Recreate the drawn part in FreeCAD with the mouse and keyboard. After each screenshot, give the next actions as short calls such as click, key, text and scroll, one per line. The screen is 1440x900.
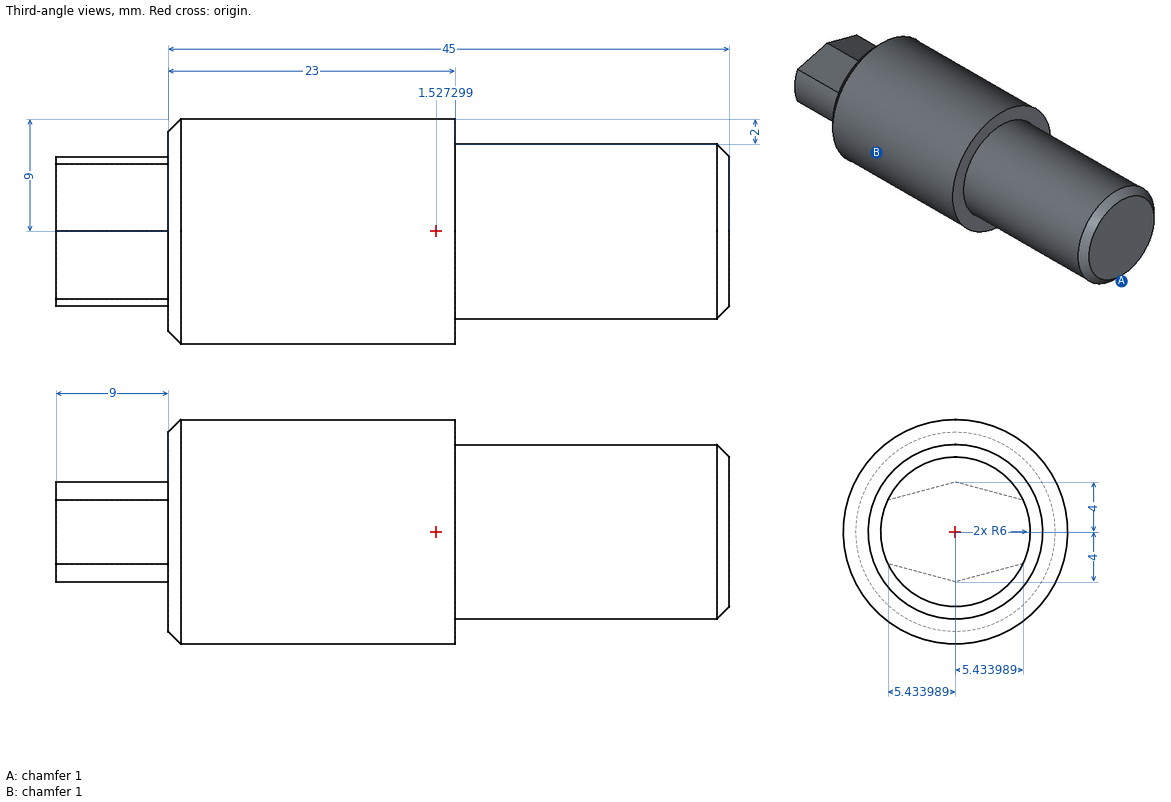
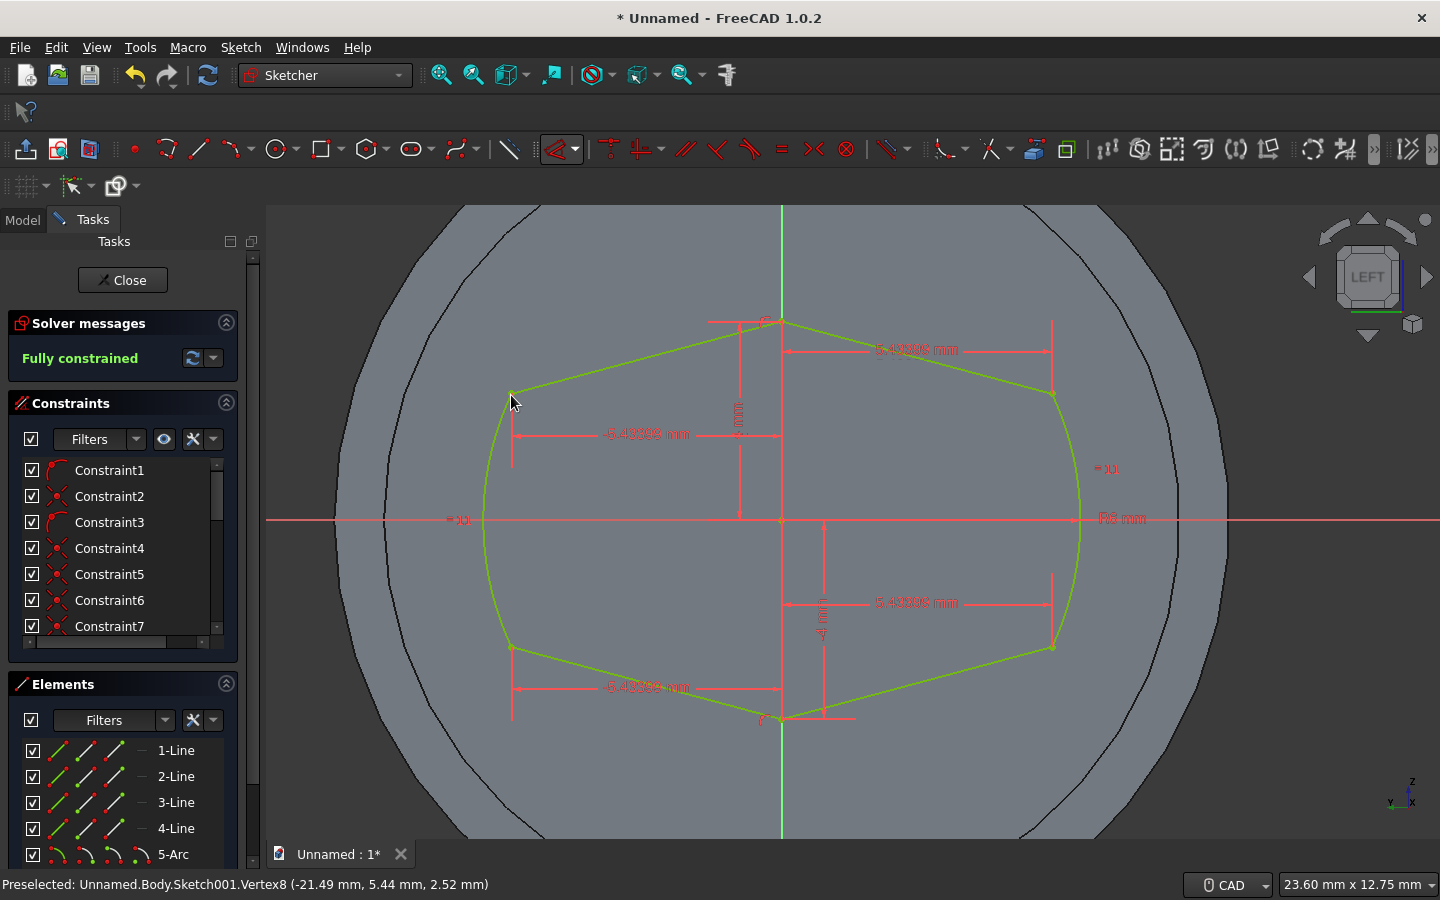
click(123, 280)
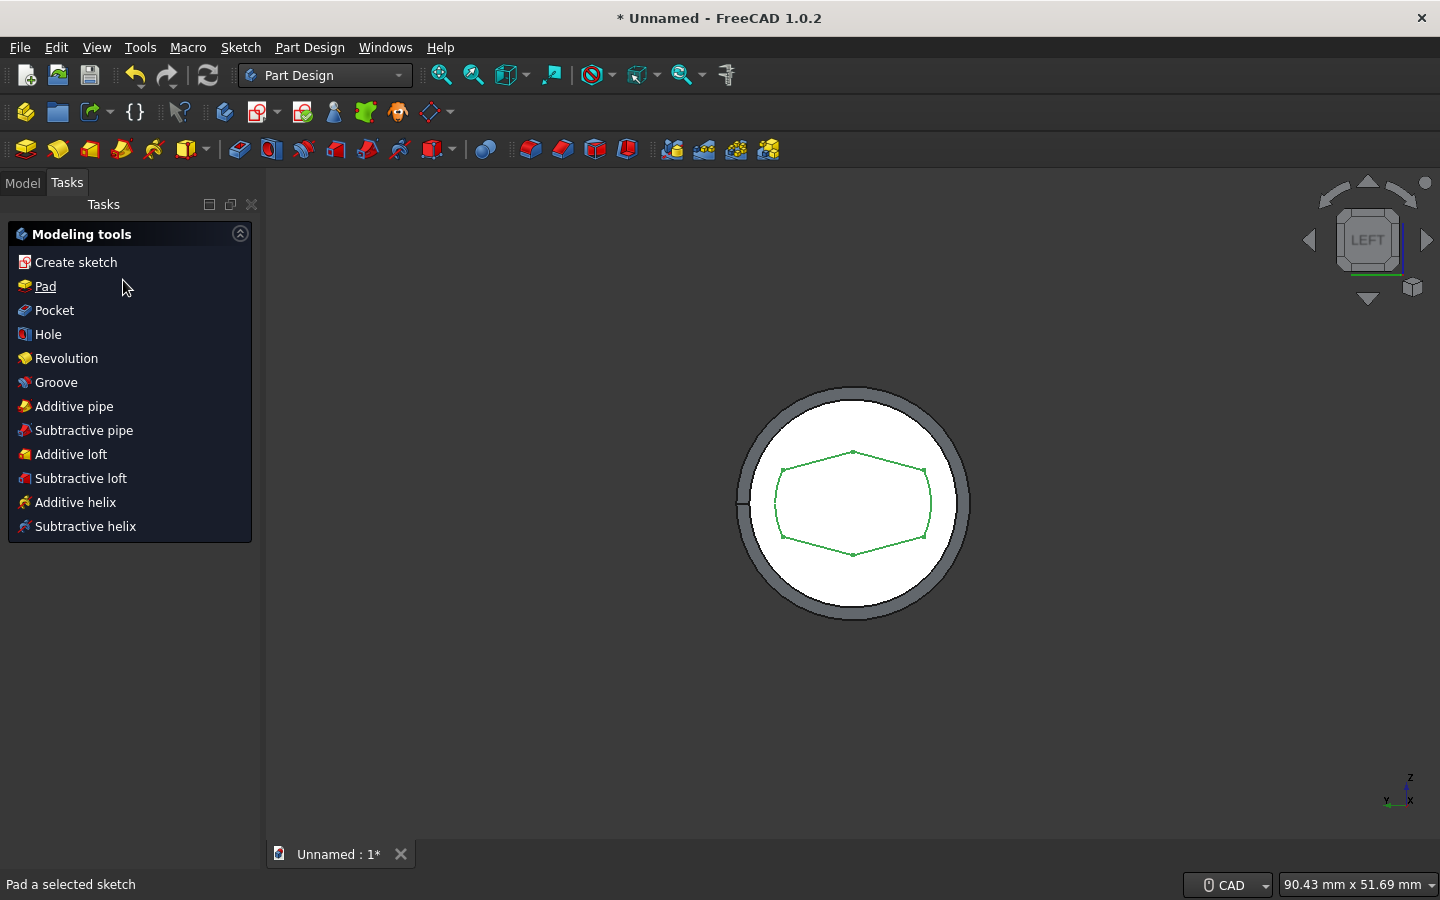
click(26, 150)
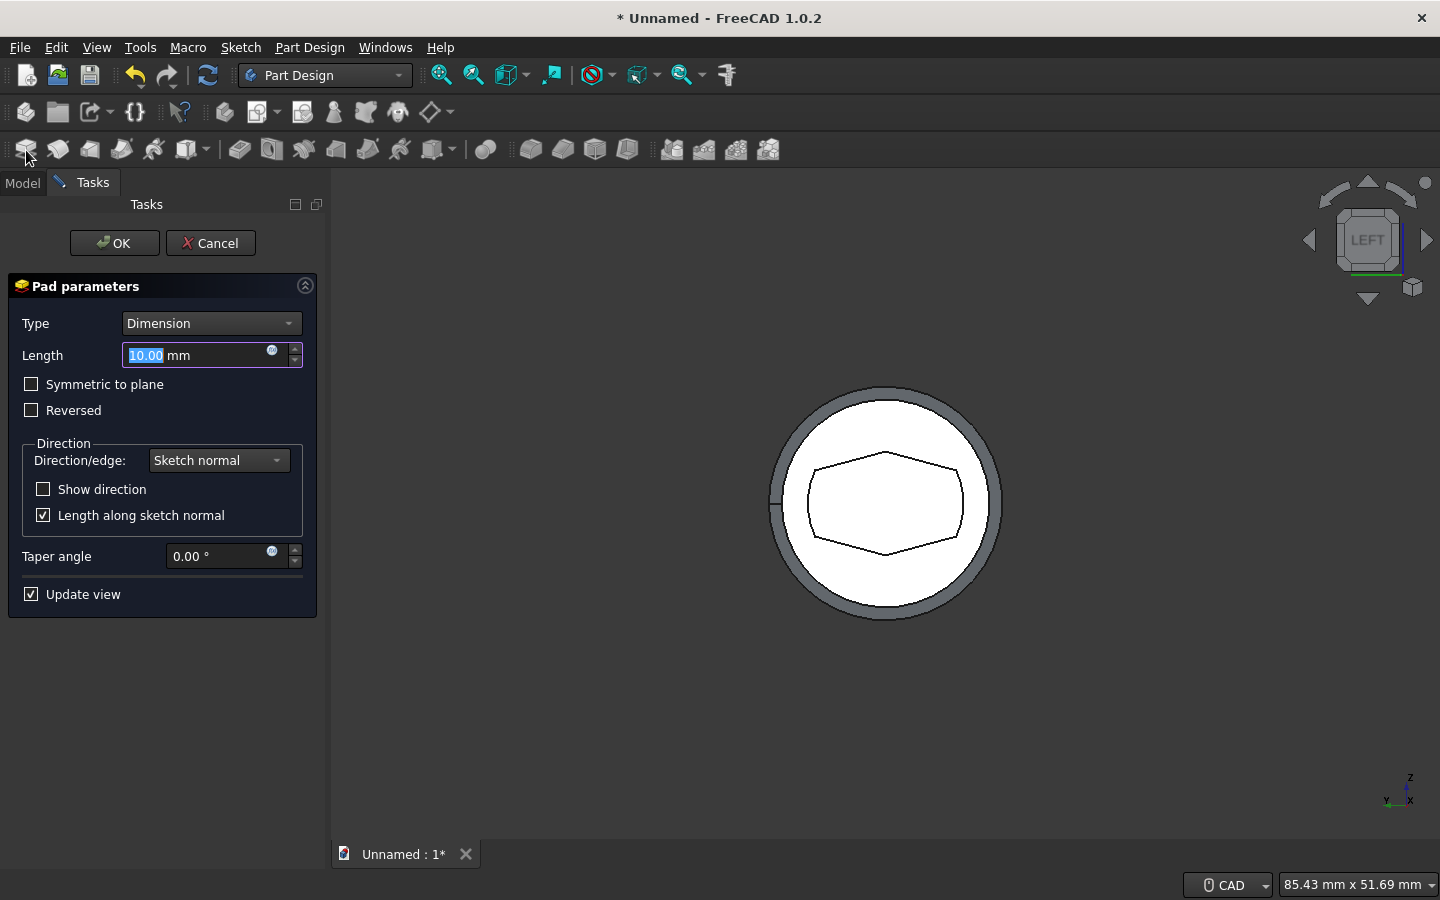
text(9)
key(Tab)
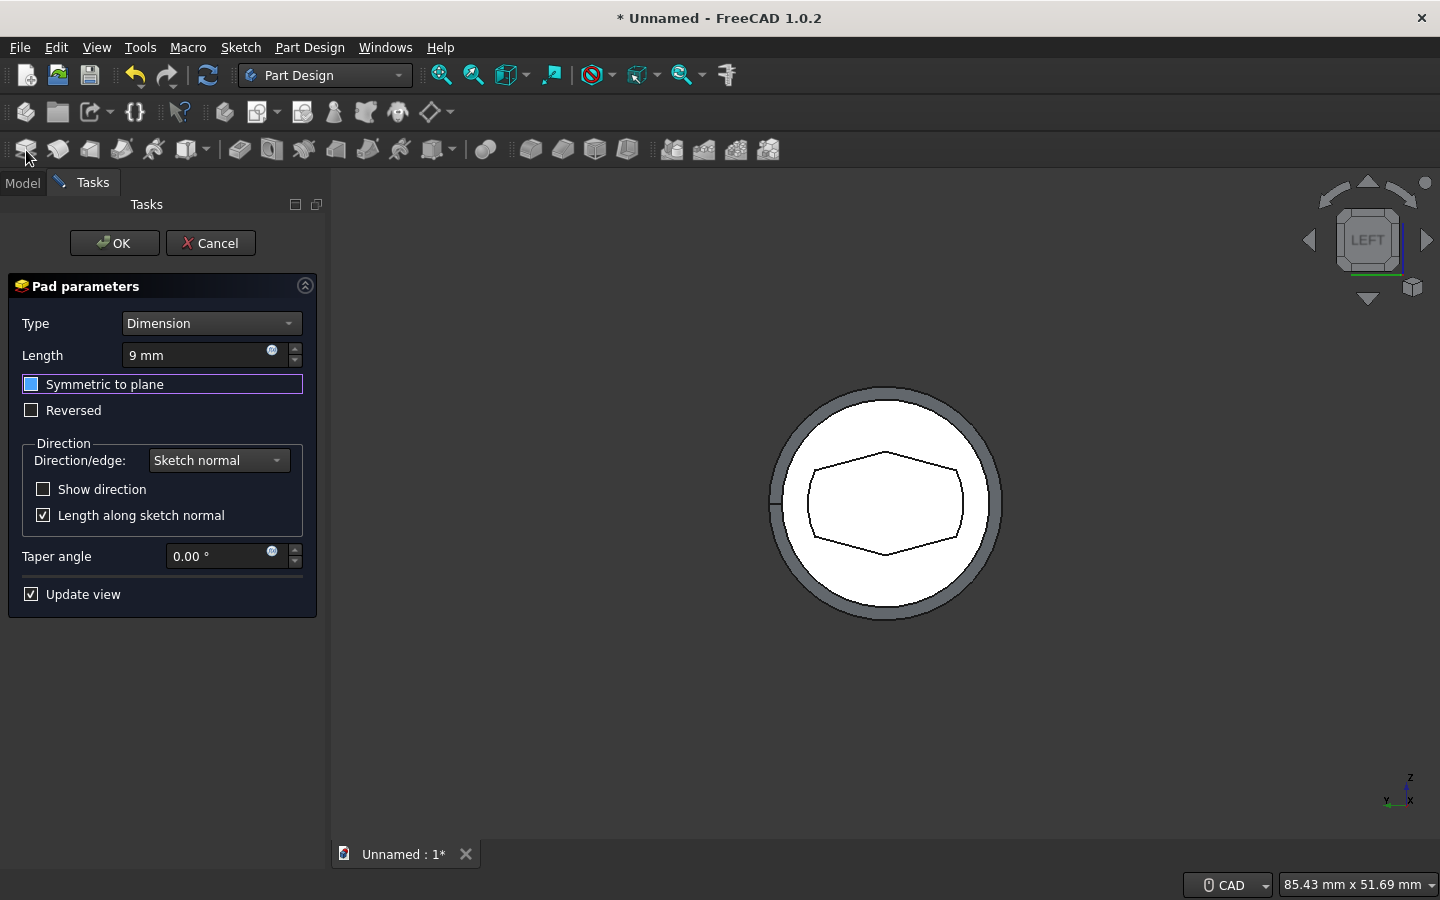
click(115, 243)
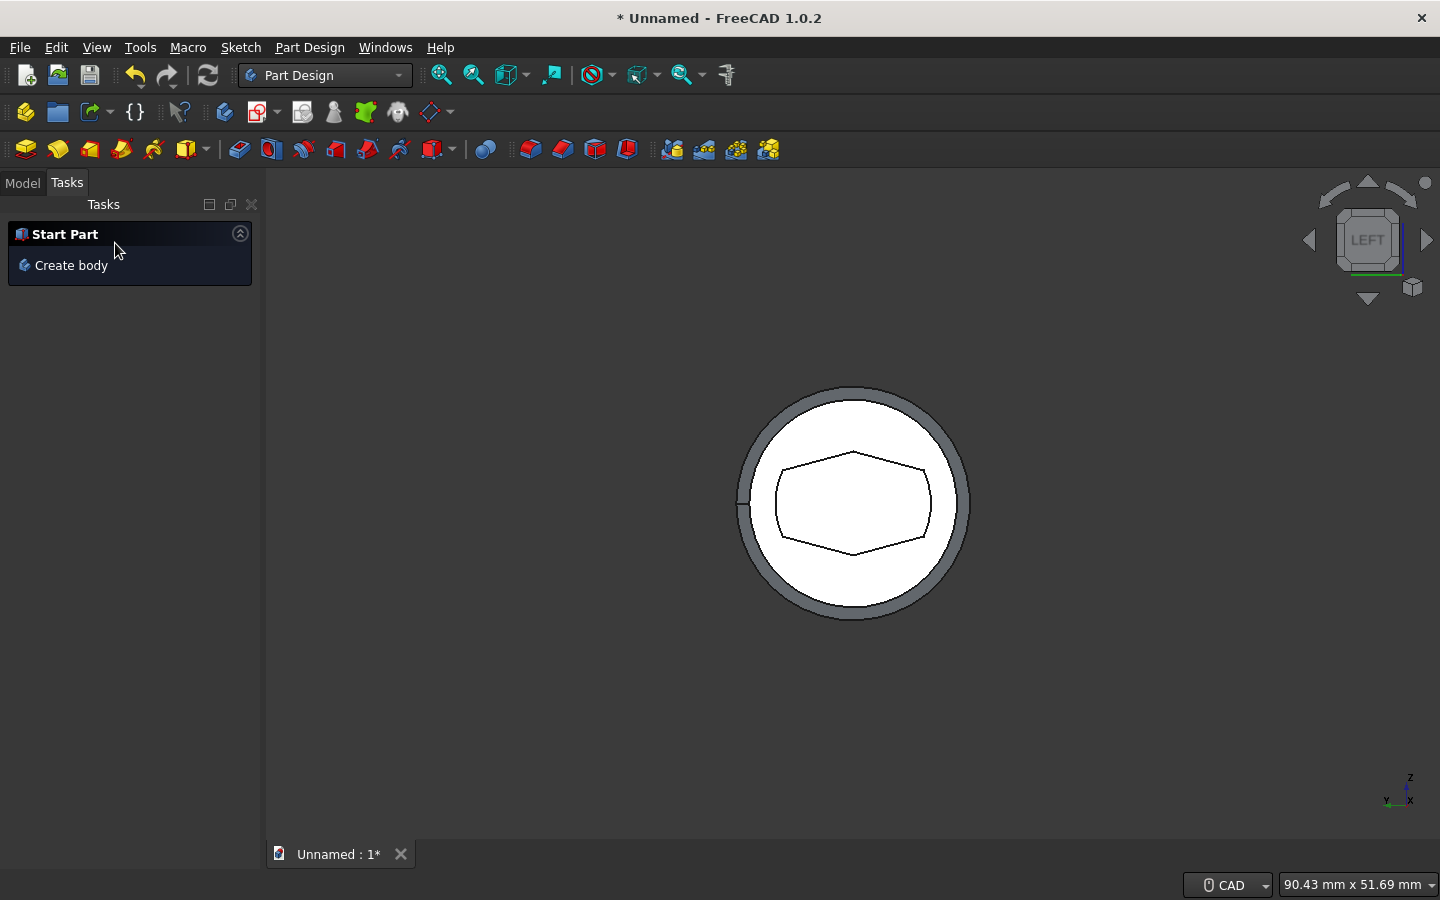
key(0)